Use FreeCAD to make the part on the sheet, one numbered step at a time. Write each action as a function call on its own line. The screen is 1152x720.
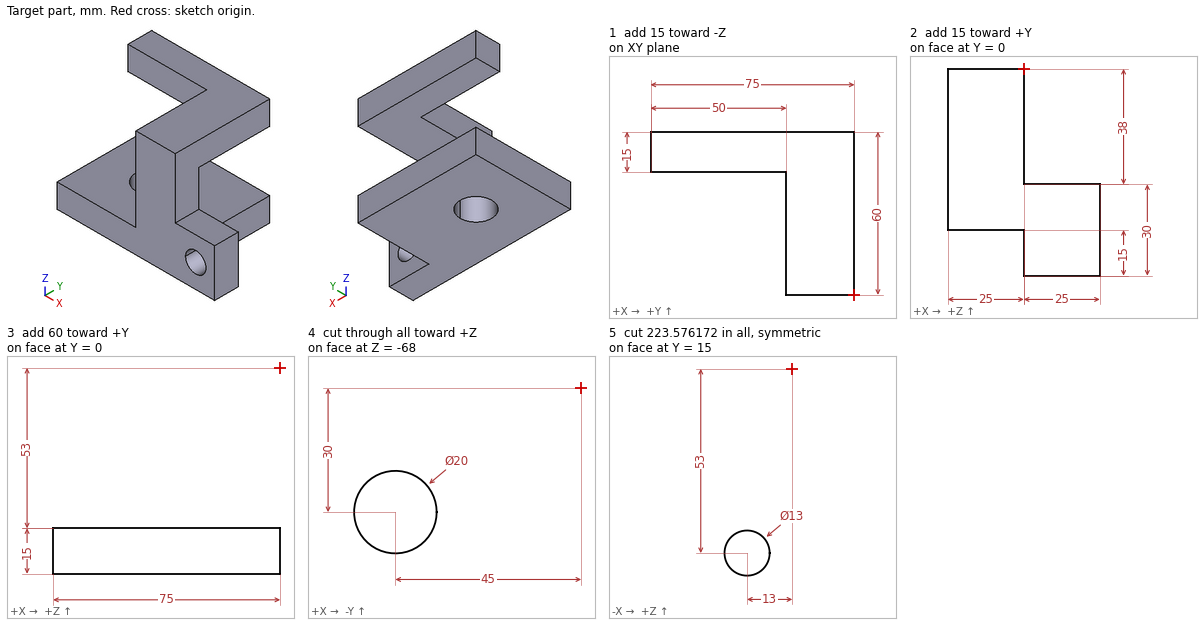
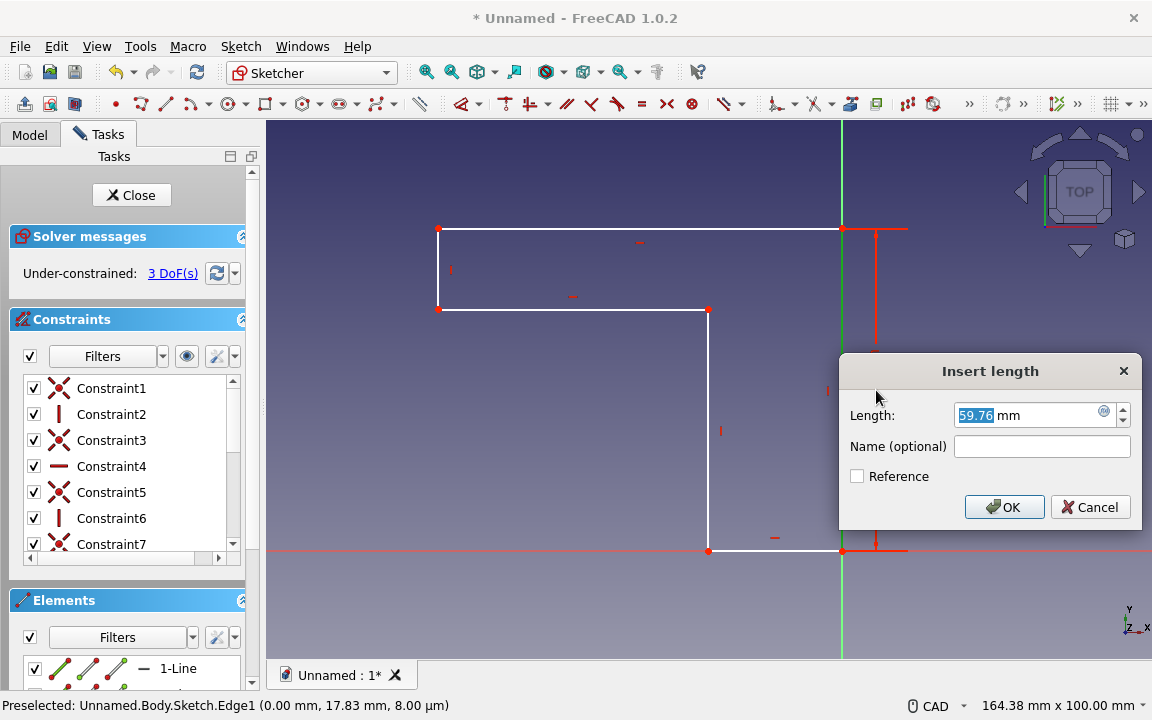
text(60)
key(Return)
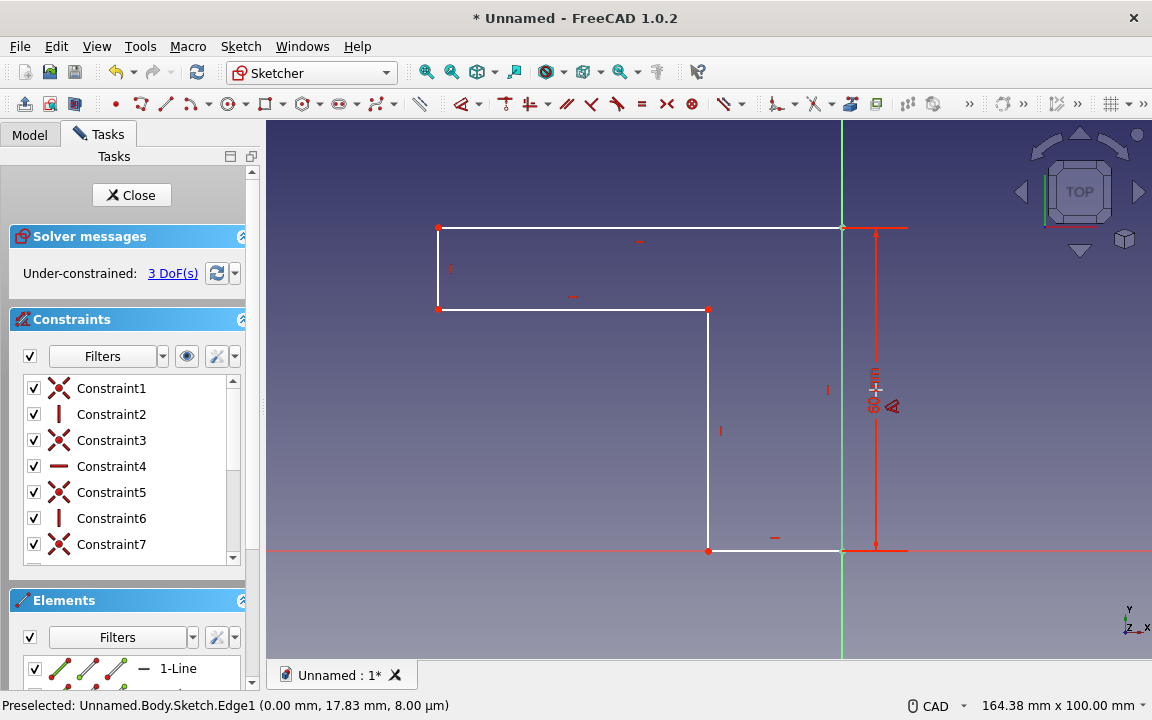
click(721, 228)
click(640, 194)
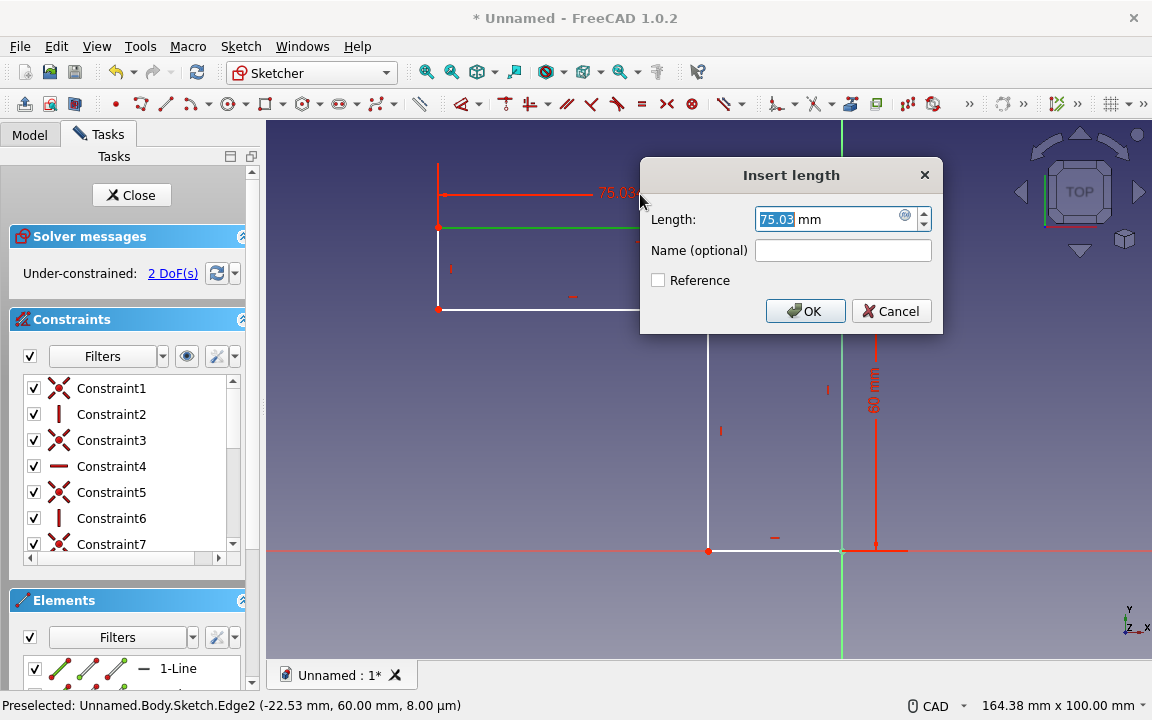
text(75)
key(Return)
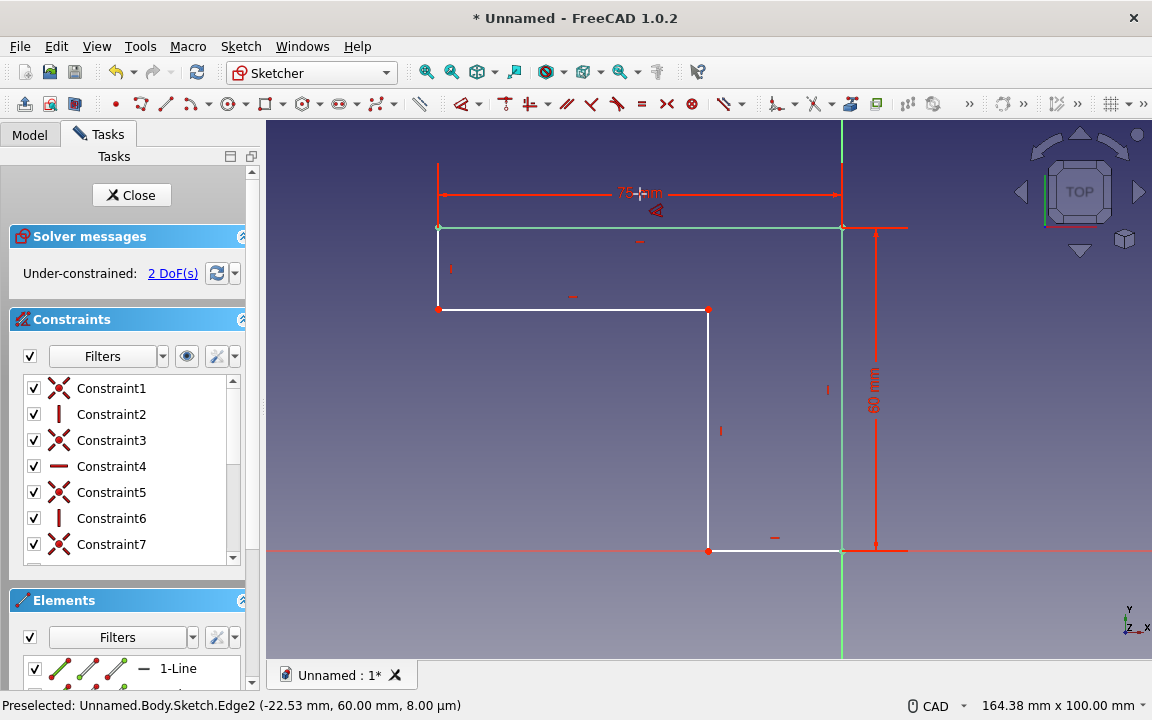
click(438, 252)
click(404, 269)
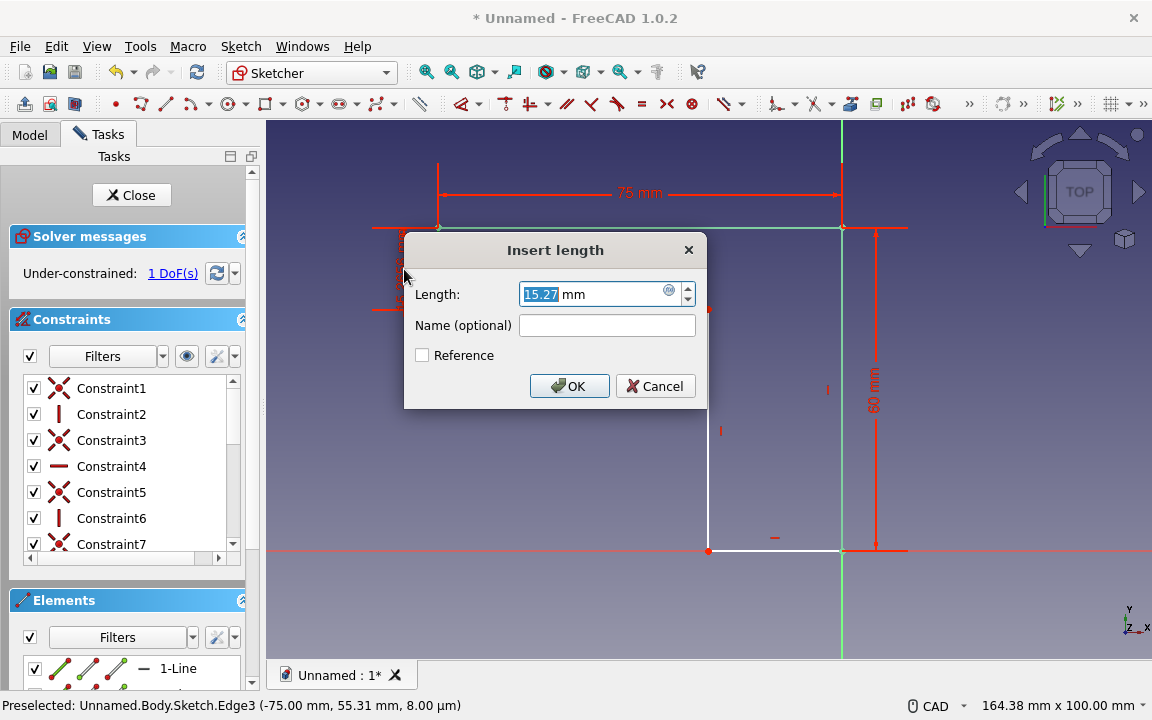
text(15)
key(Return)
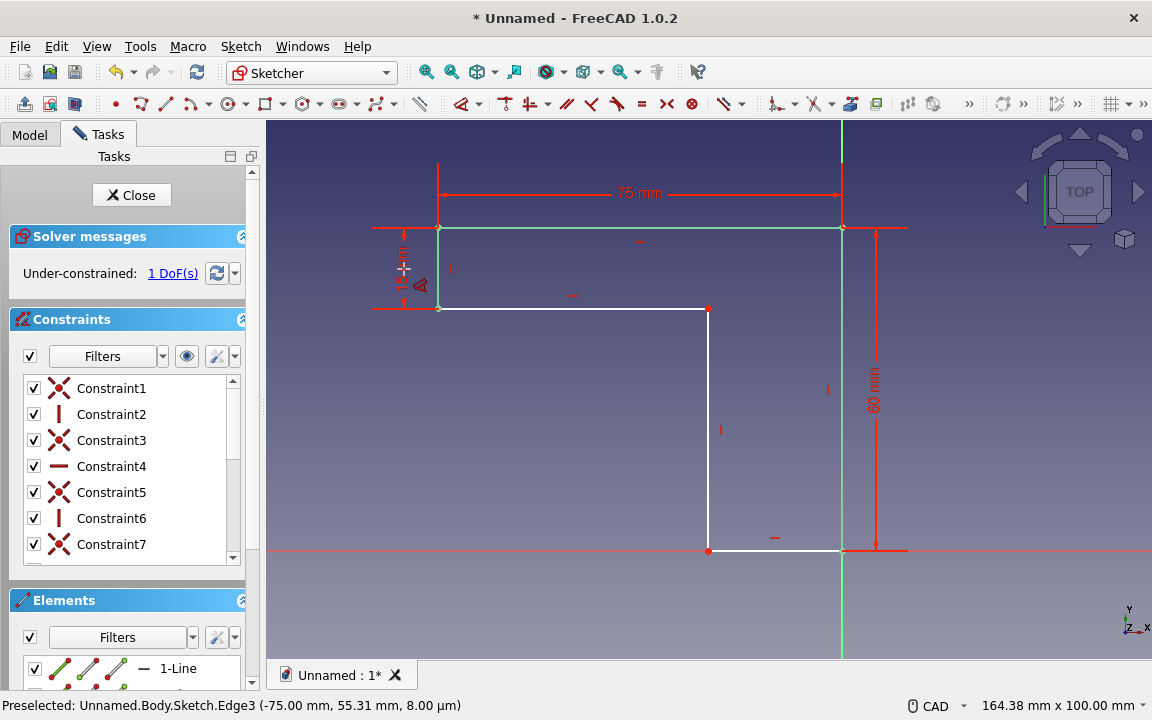
click(519, 309)
click(573, 275)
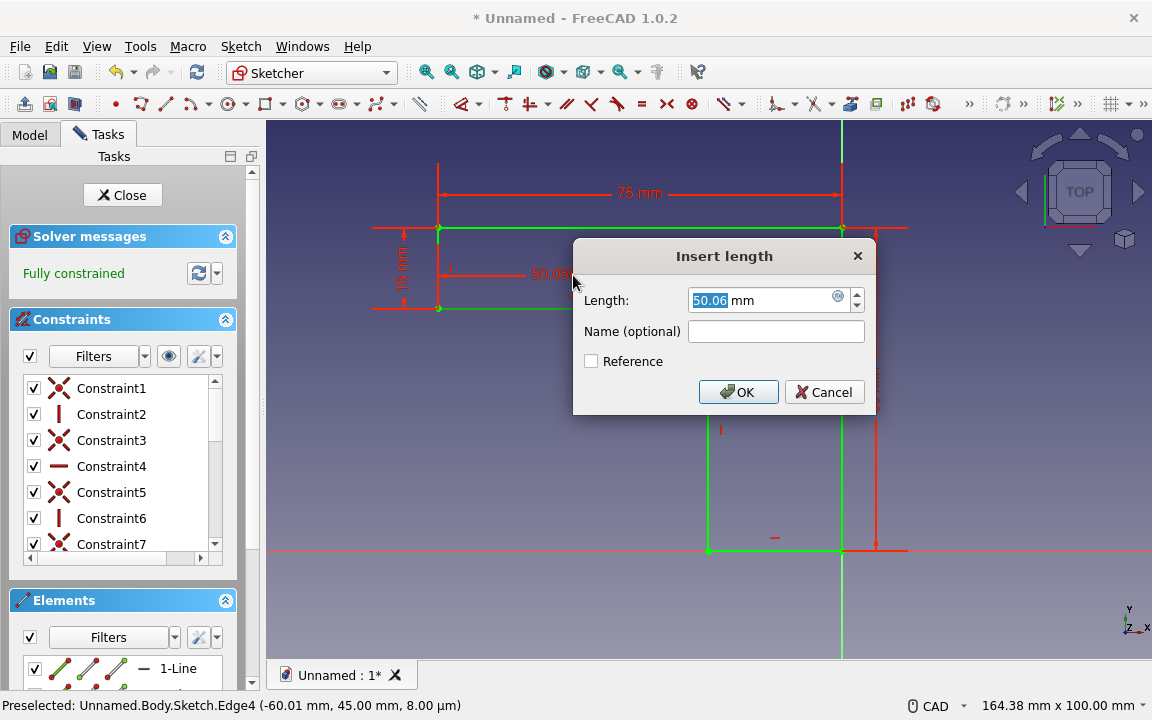
text(50)
key(Return)
key(Escape)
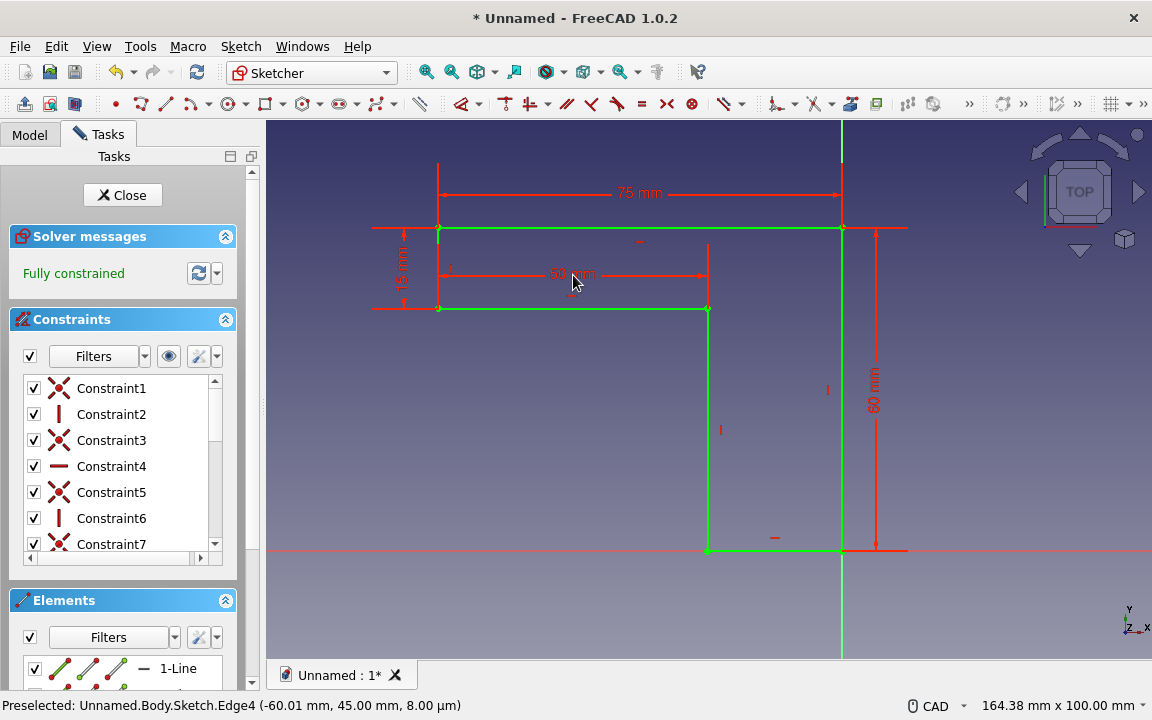
click(123, 195)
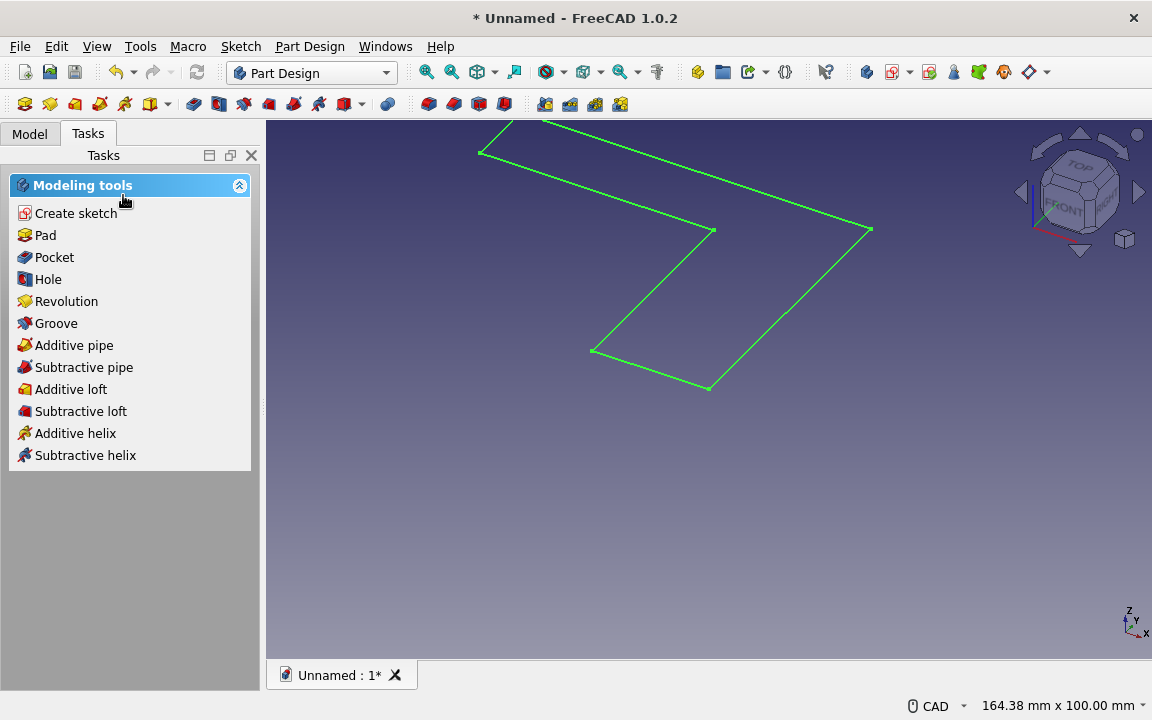
click(25, 104)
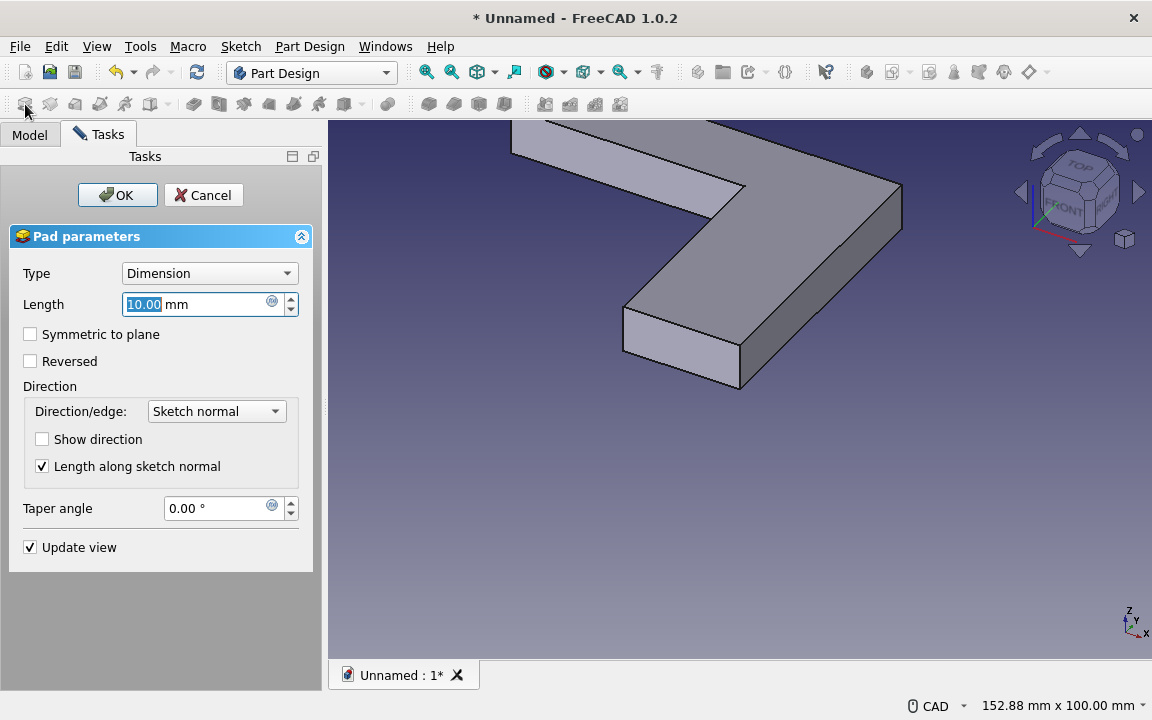
text(15)
key(Tab)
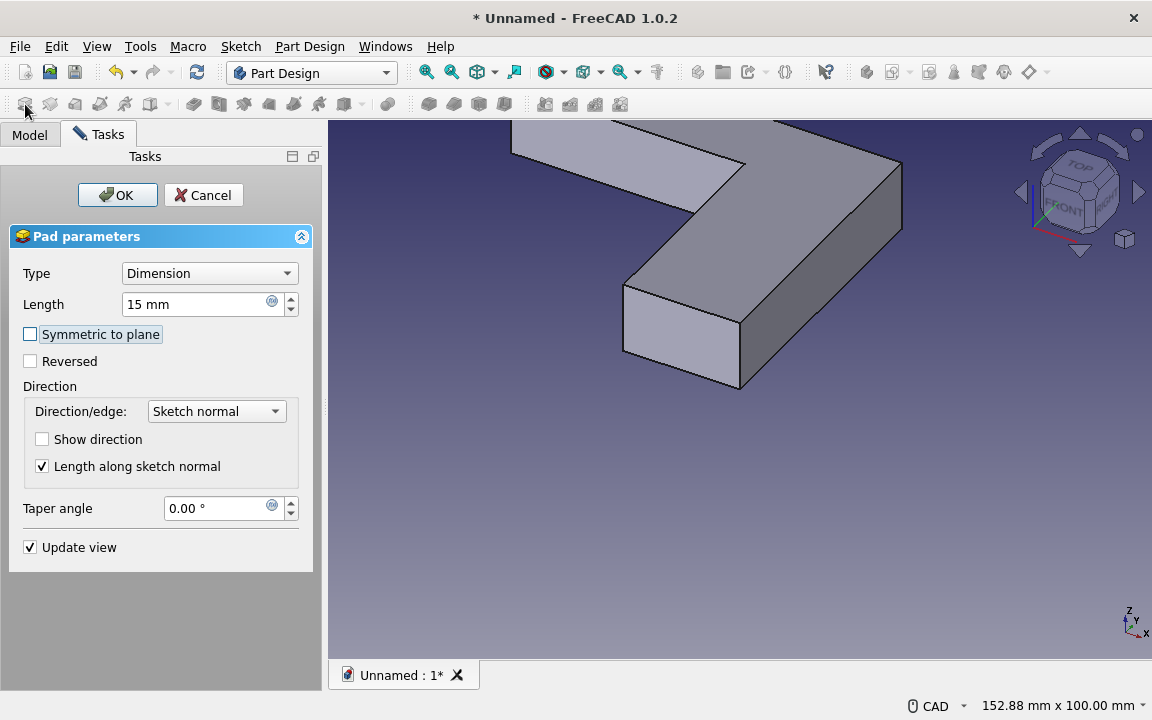
click(31, 361)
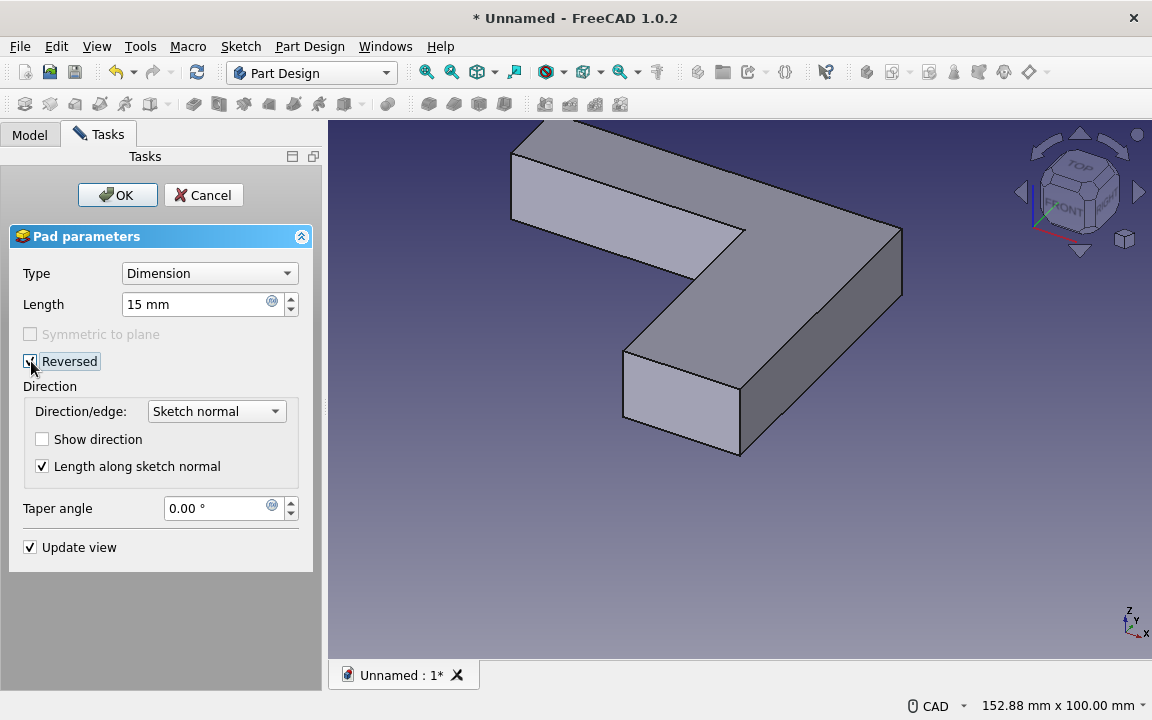
click(118, 195)